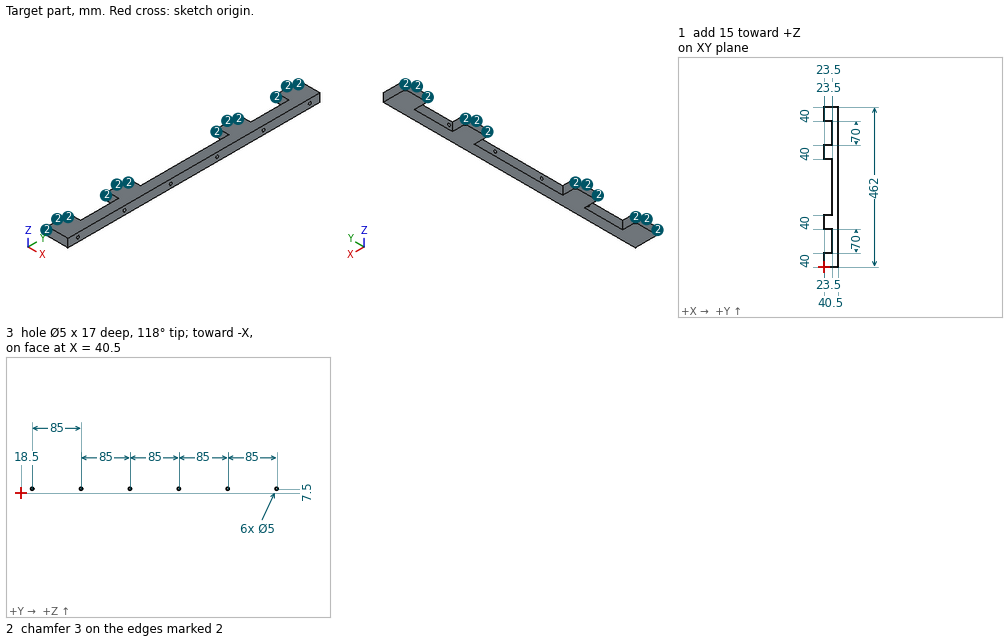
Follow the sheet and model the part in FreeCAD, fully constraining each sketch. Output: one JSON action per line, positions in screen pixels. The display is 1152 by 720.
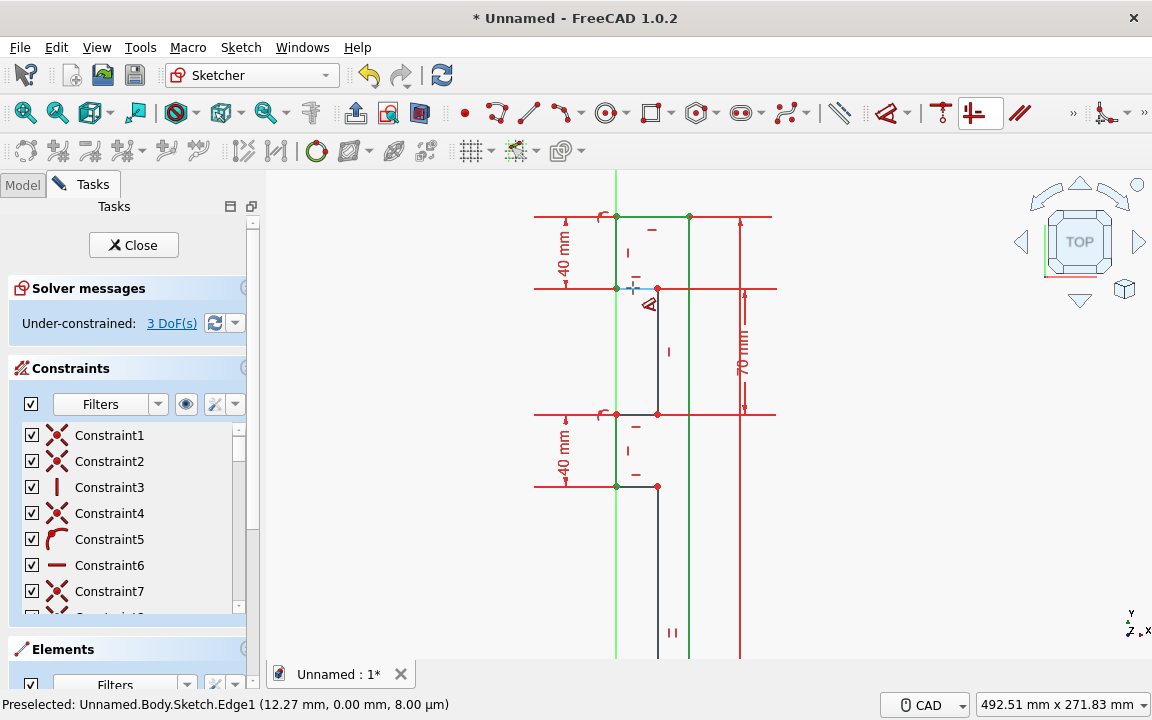
{"action": "left_click", "coordinate": [633, 289]}
{"action": "left_click", "coordinate": [637, 255]}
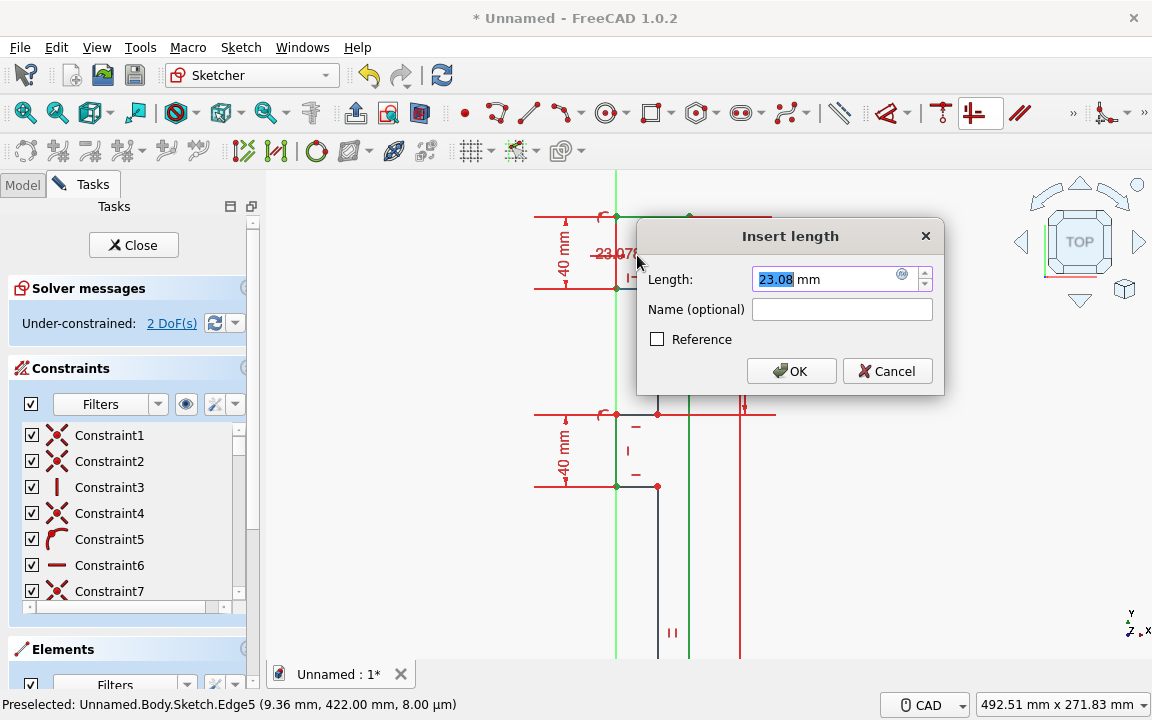
{"action": "type", "text": "23.5"}
{"action": "key", "text": "Return"}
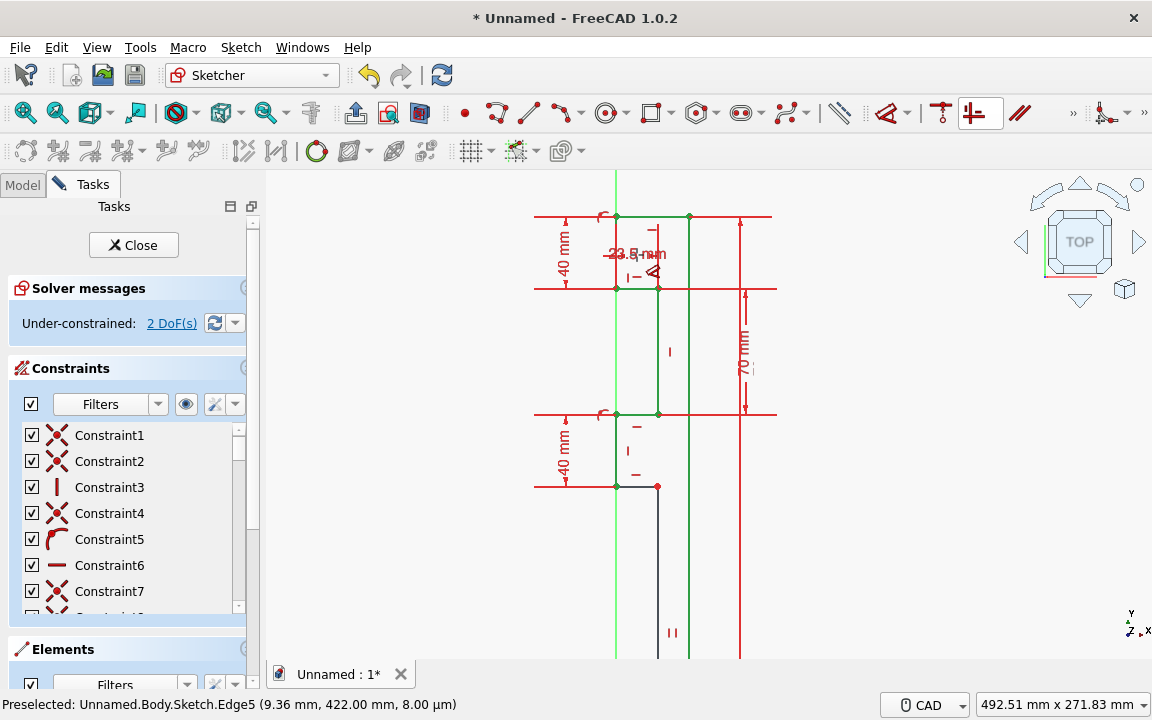
{"action": "left_click", "coordinate": [629, 487]}
{"action": "left_click", "coordinate": [637, 453]}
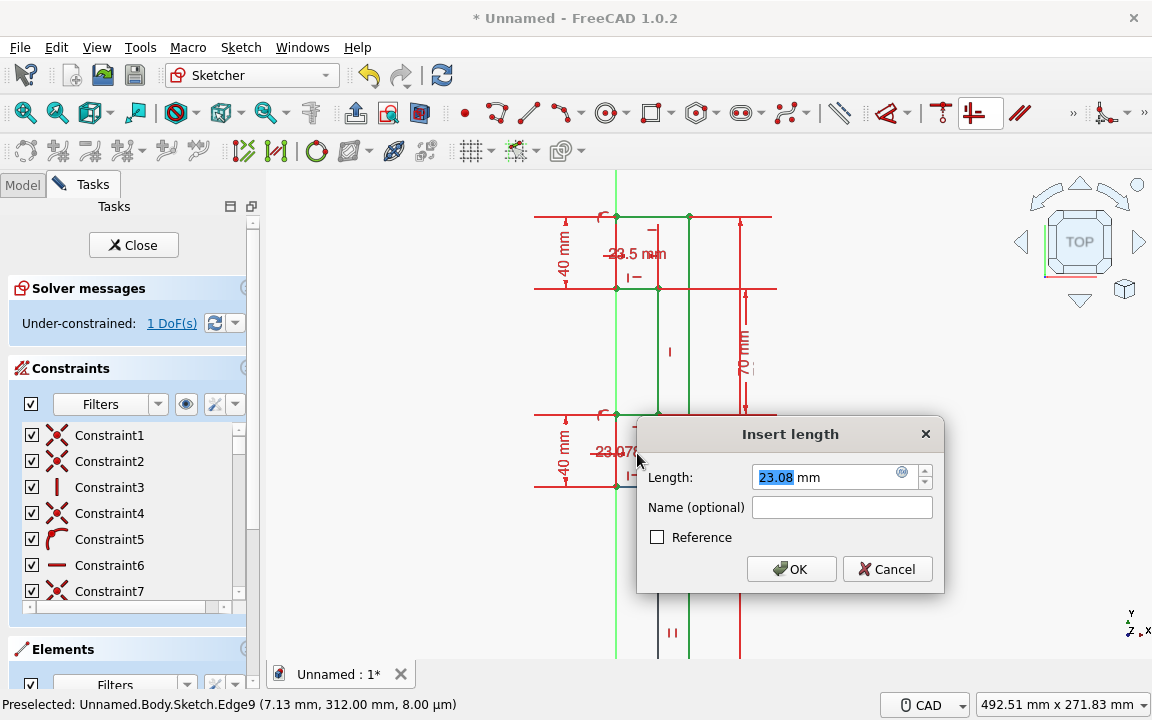
{"action": "type", "text": "23.5"}
{"action": "key", "text": "Return"}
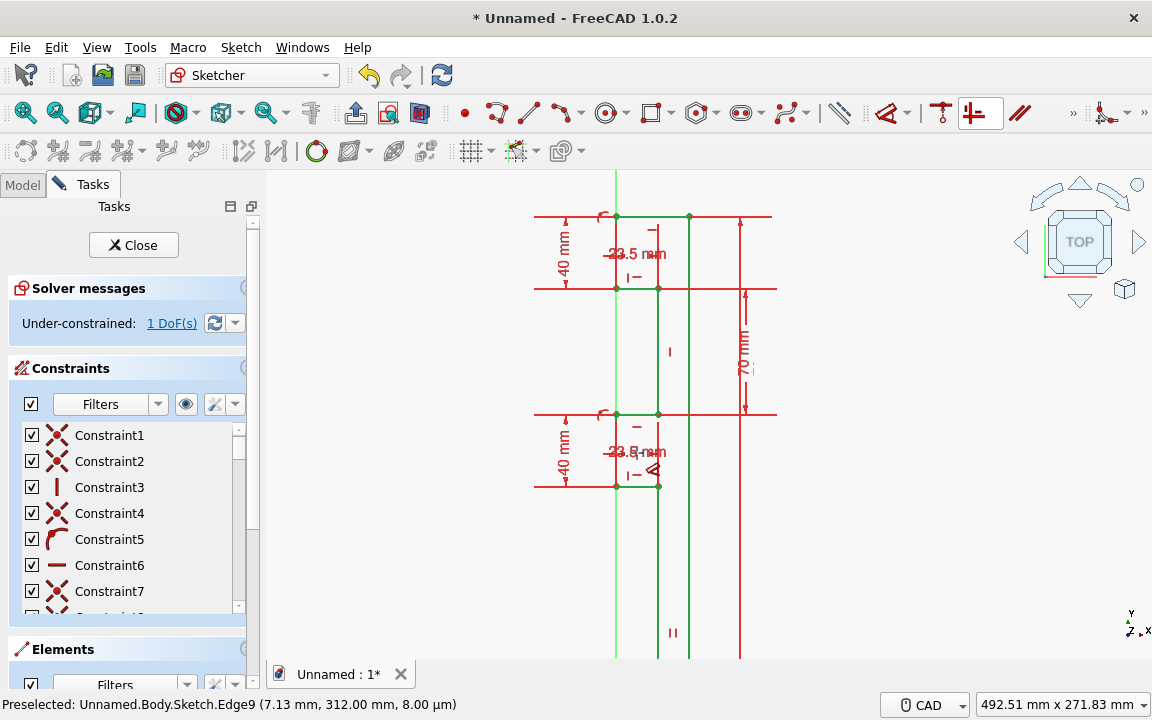
{"action": "scroll", "coordinate": [633, 288], "scroll_direction": "down", "scroll_amount": 5}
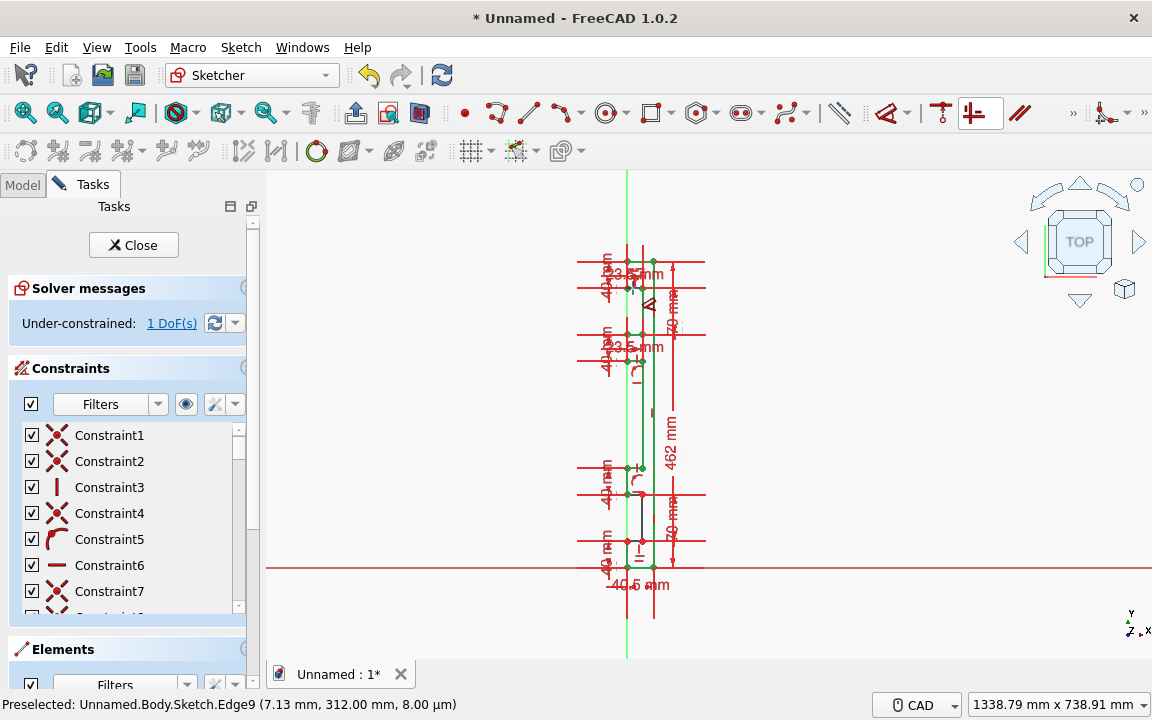
{"action": "scroll", "coordinate": [632, 495], "scroll_direction": "up", "scroll_amount": 6}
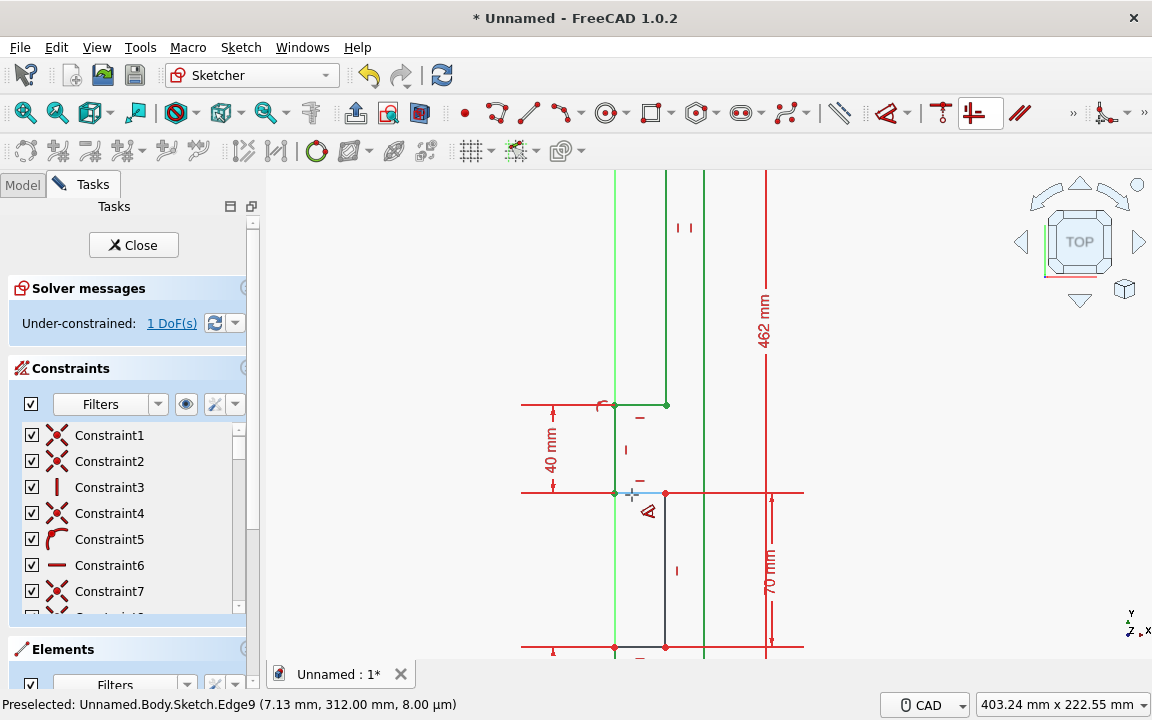
{"action": "left_click", "coordinate": [630, 493]}
{"action": "left_click", "coordinate": [640, 527]}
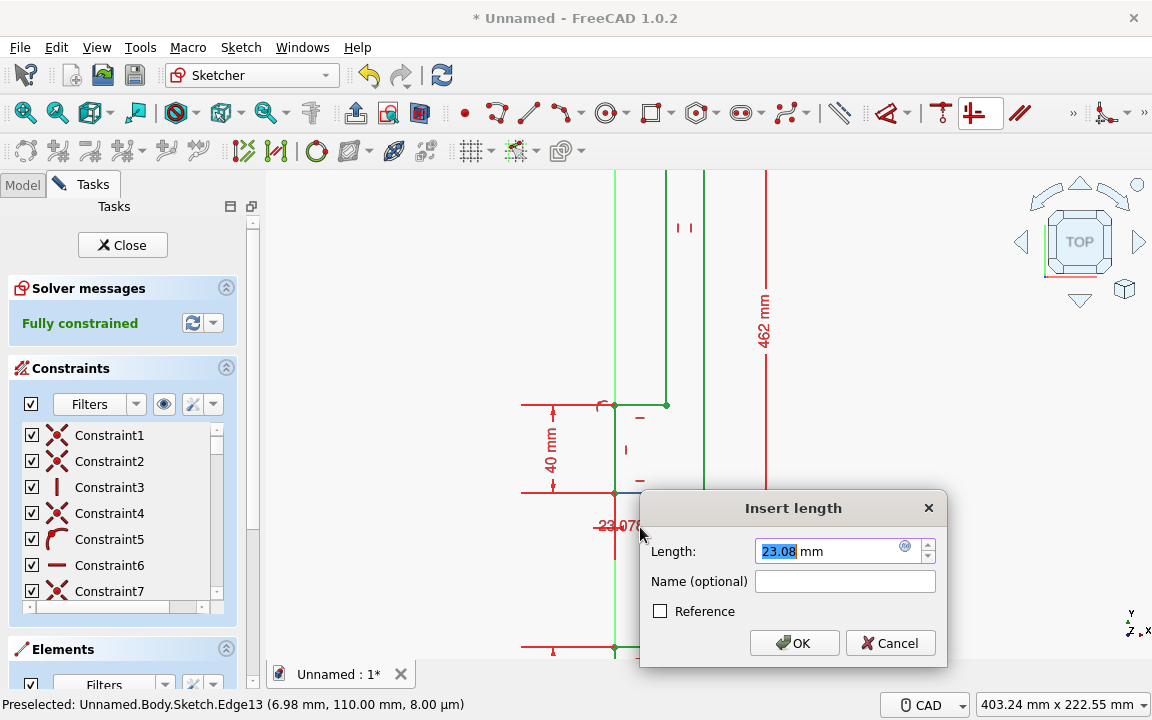
{"action": "type", "text": "23.5"}
{"action": "key", "text": "Return"}
{"action": "key", "text": "Escape"}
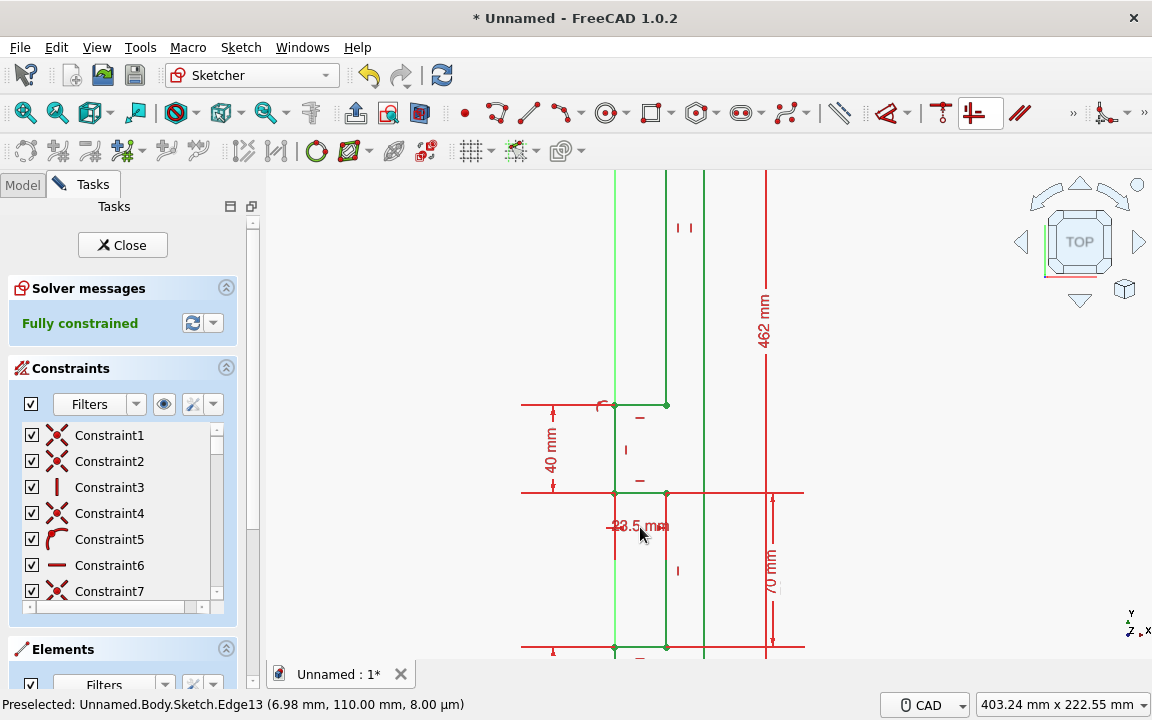
{"action": "left_click", "coordinate": [123, 245]}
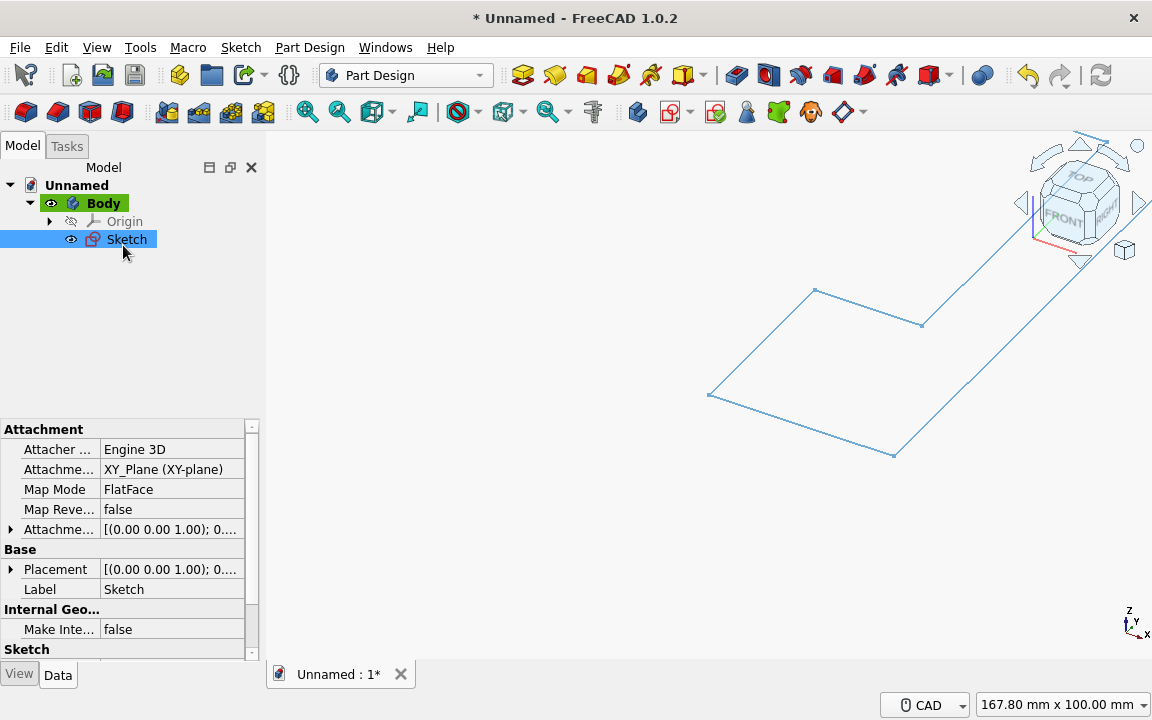
{"action": "left_click", "coordinate": [524, 76]}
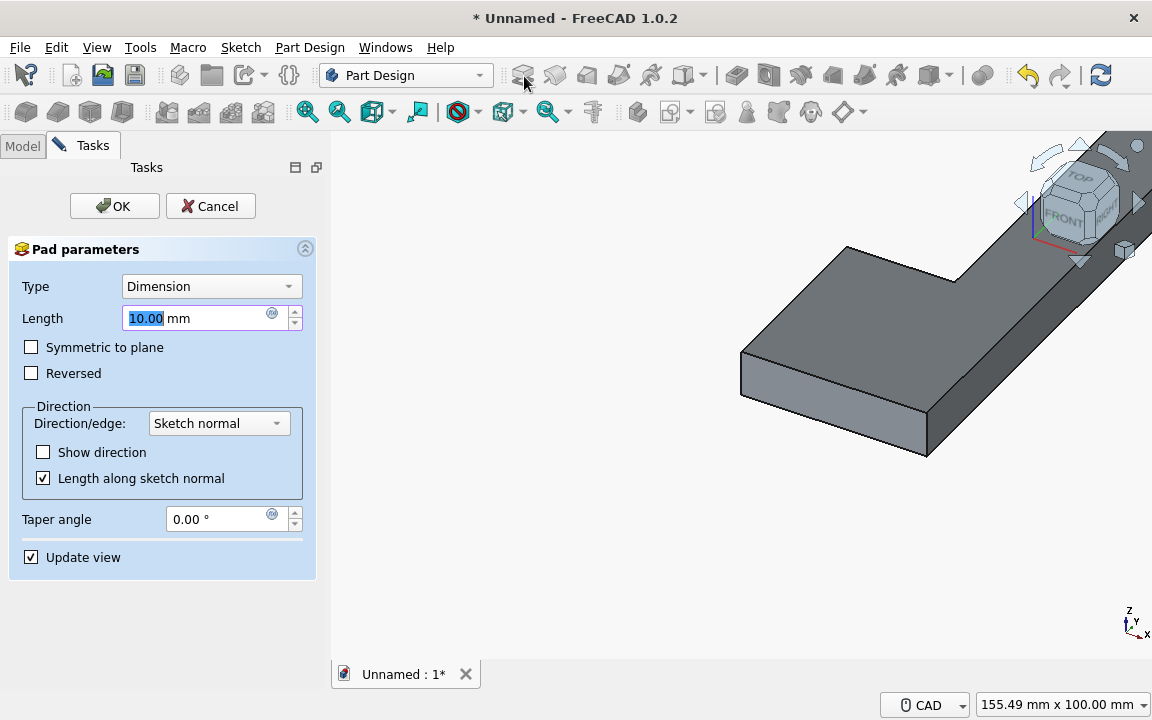
{"action": "type", "text": "15"}
{"action": "key", "text": "Tab"}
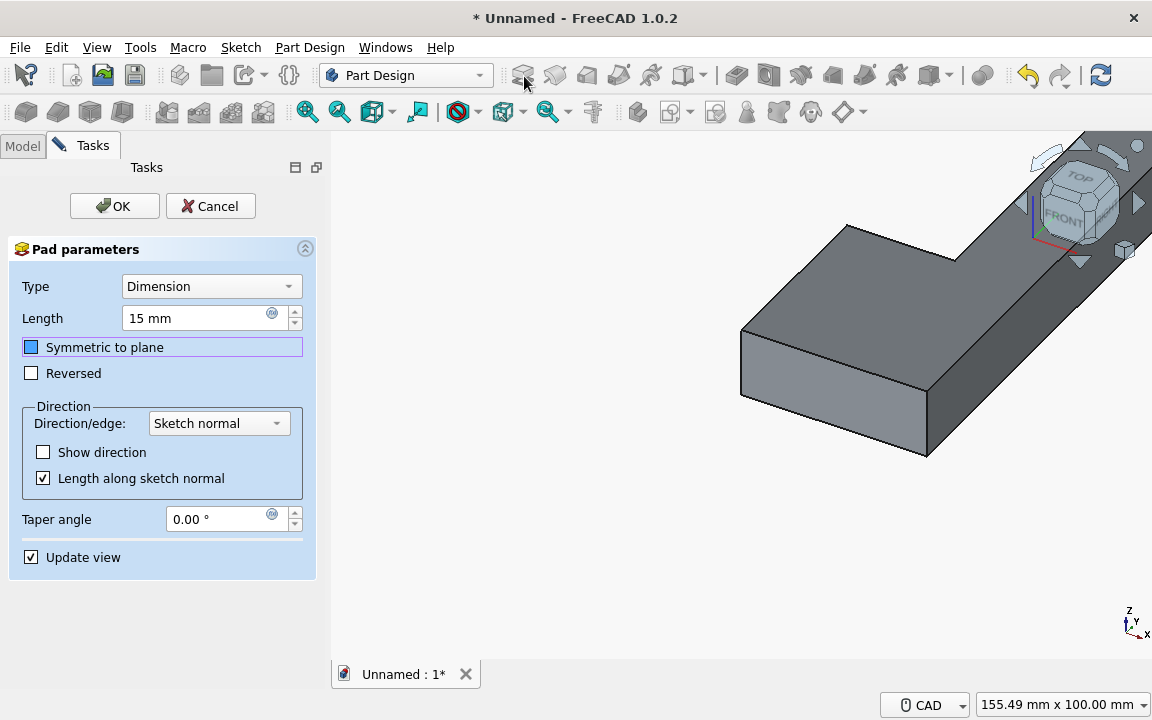
{"action": "left_click", "coordinate": [115, 206]}